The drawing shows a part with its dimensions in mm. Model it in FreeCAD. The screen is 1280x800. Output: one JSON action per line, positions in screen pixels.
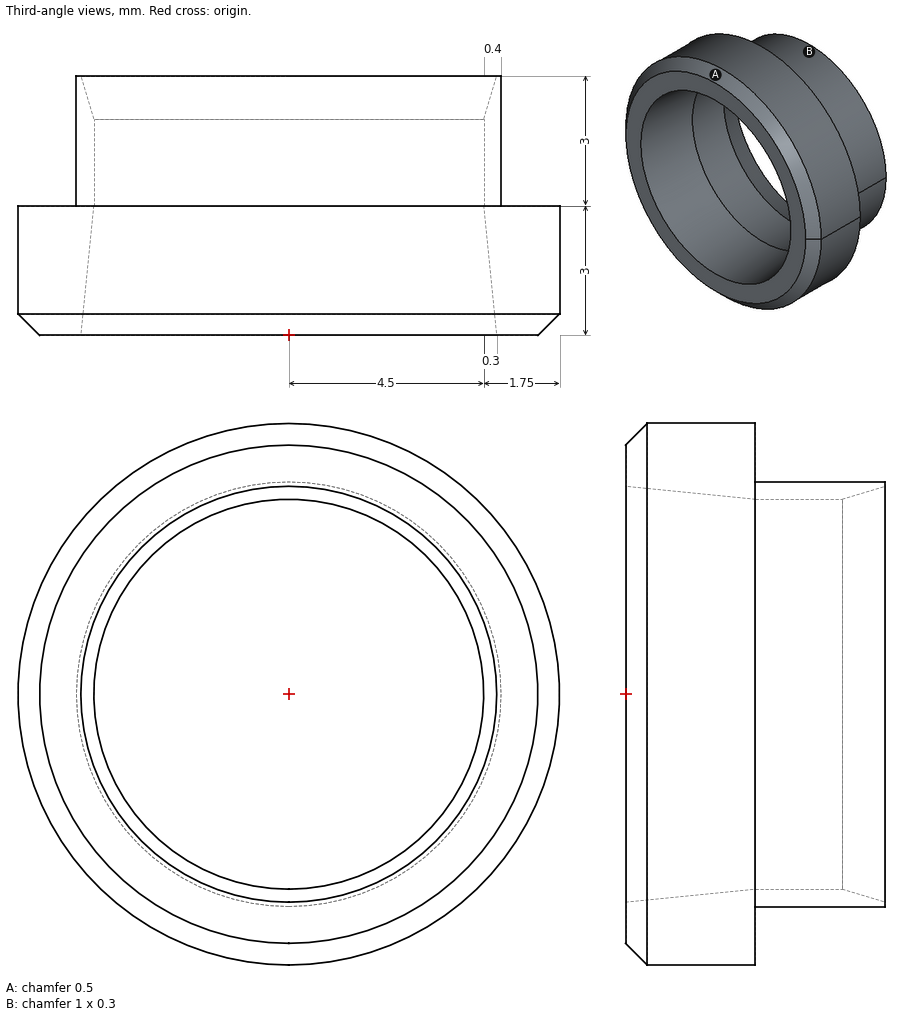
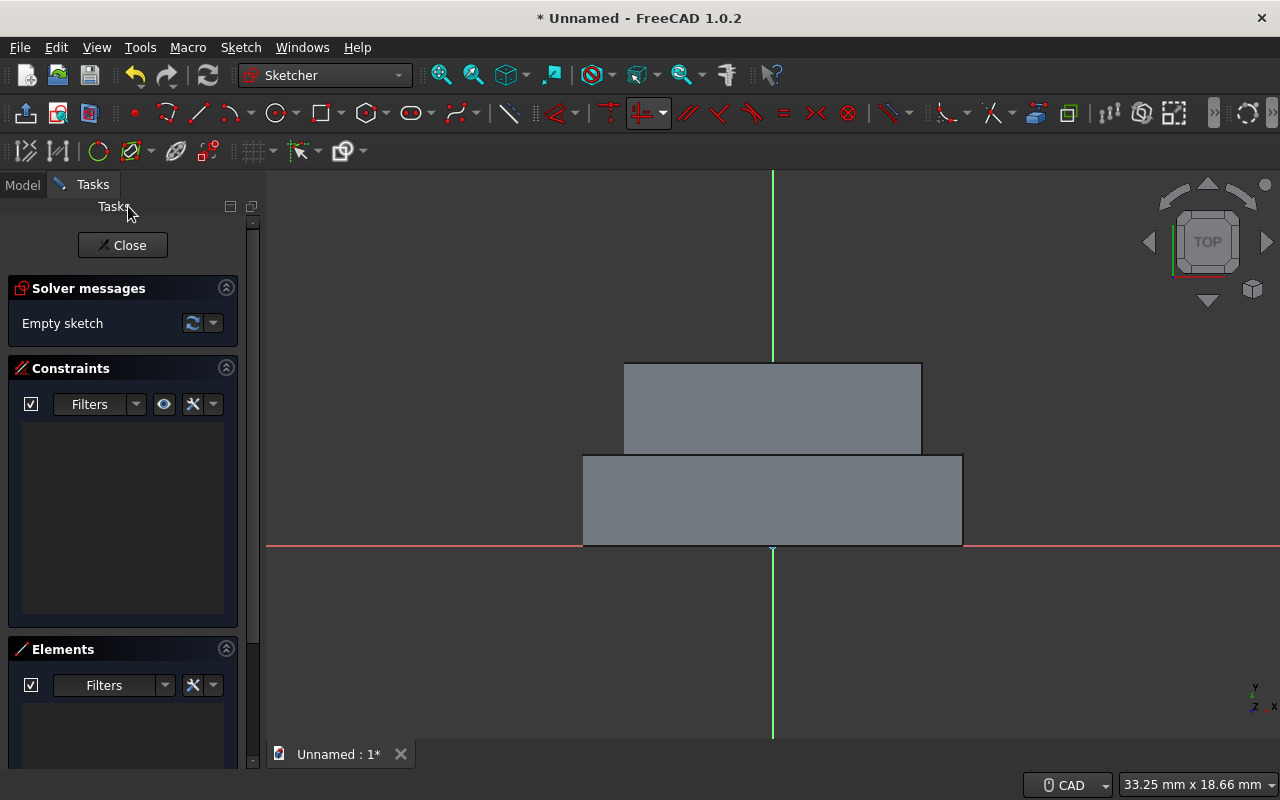
{"action": "left_click", "coordinate": [90, 114]}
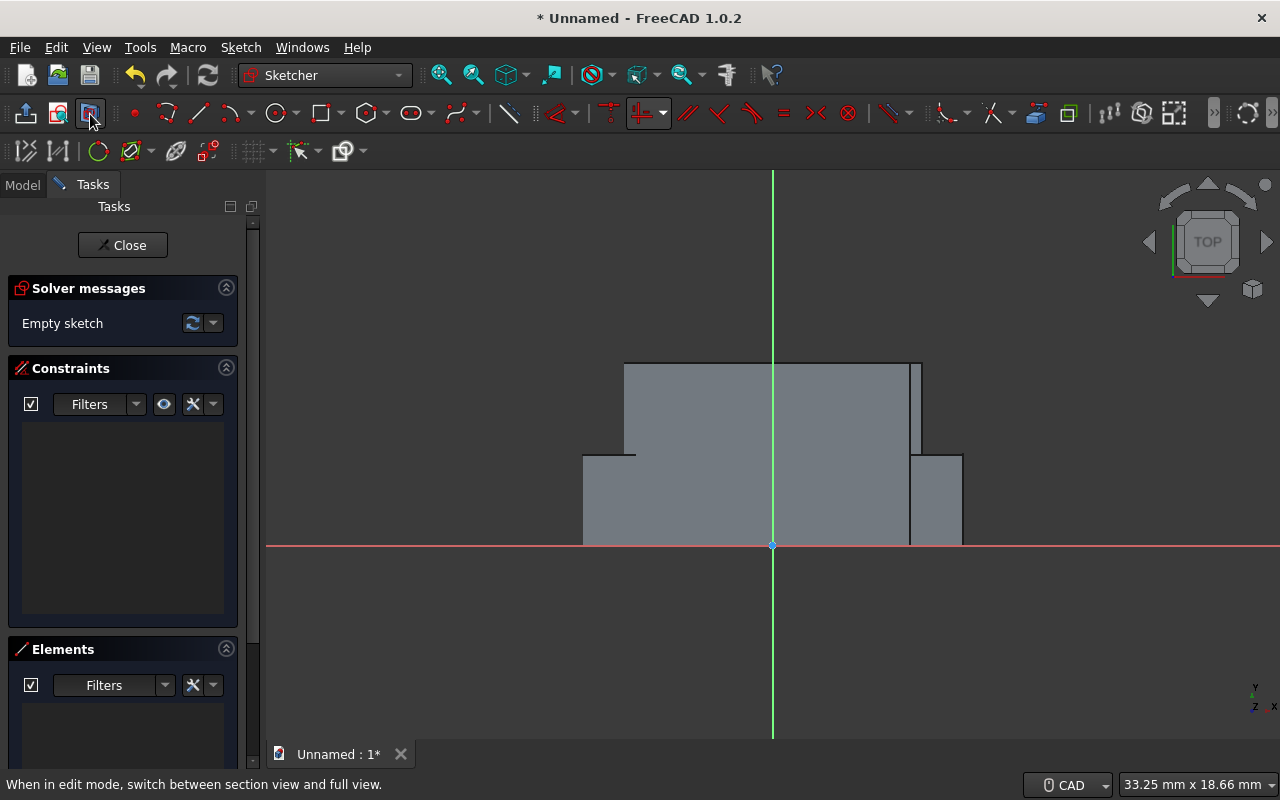
{"action": "scroll", "coordinate": [892, 515], "scroll_direction": "up", "scroll_amount": 7}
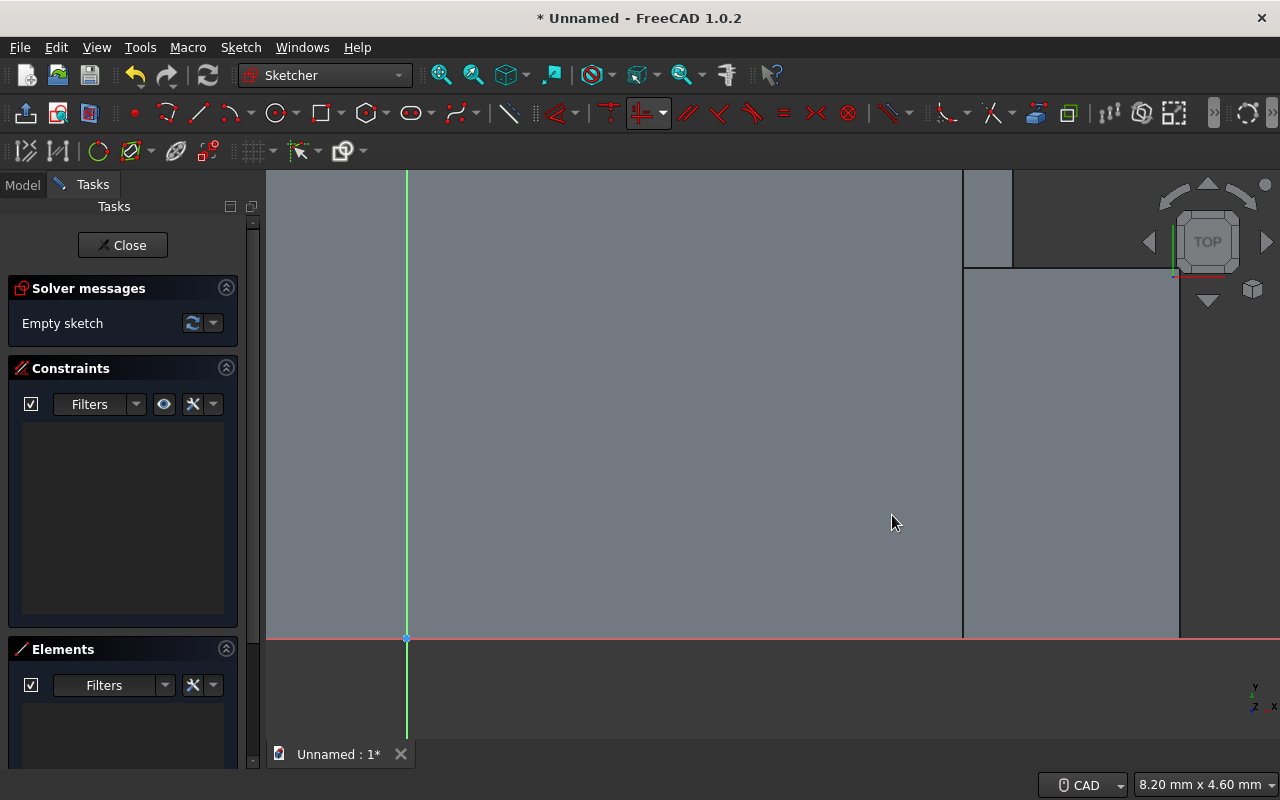
{"action": "key", "text": "g m"}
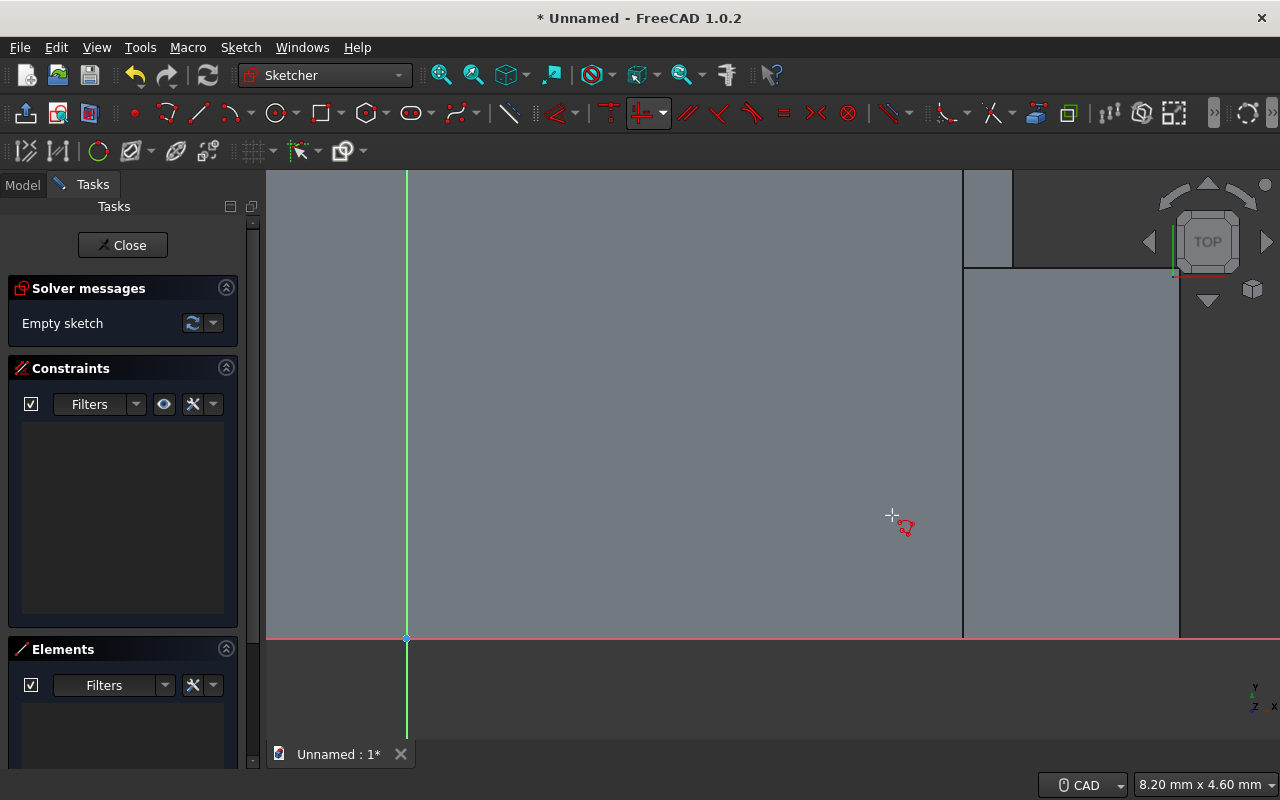
{"action": "left_click", "coordinate": [963, 639]}
{"action": "left_click", "coordinate": [1001, 630]}
{"action": "left_click", "coordinate": [963, 268]}
{"action": "left_click", "coordinate": [963, 639]}
{"action": "key", "text": "Escape"}
{"action": "key", "text": "Escape"}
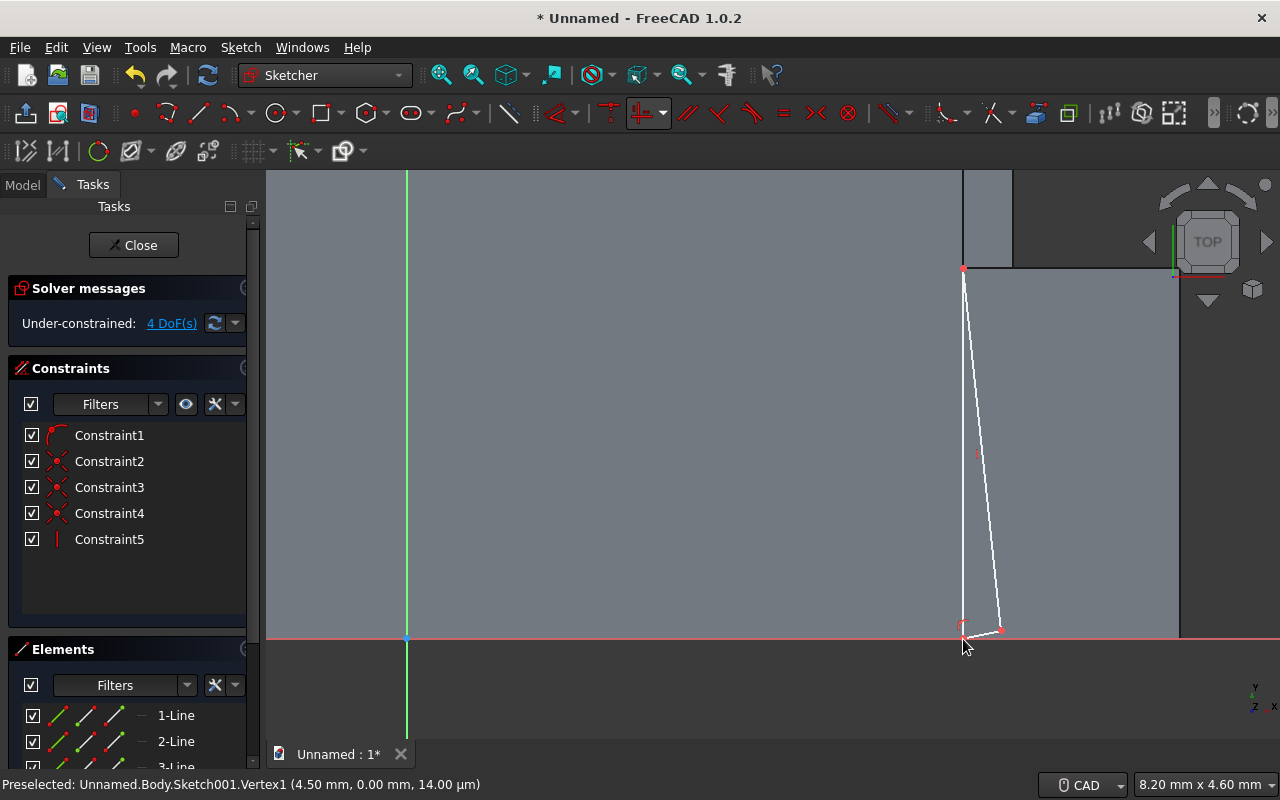
{"action": "left_click", "coordinate": [974, 636]}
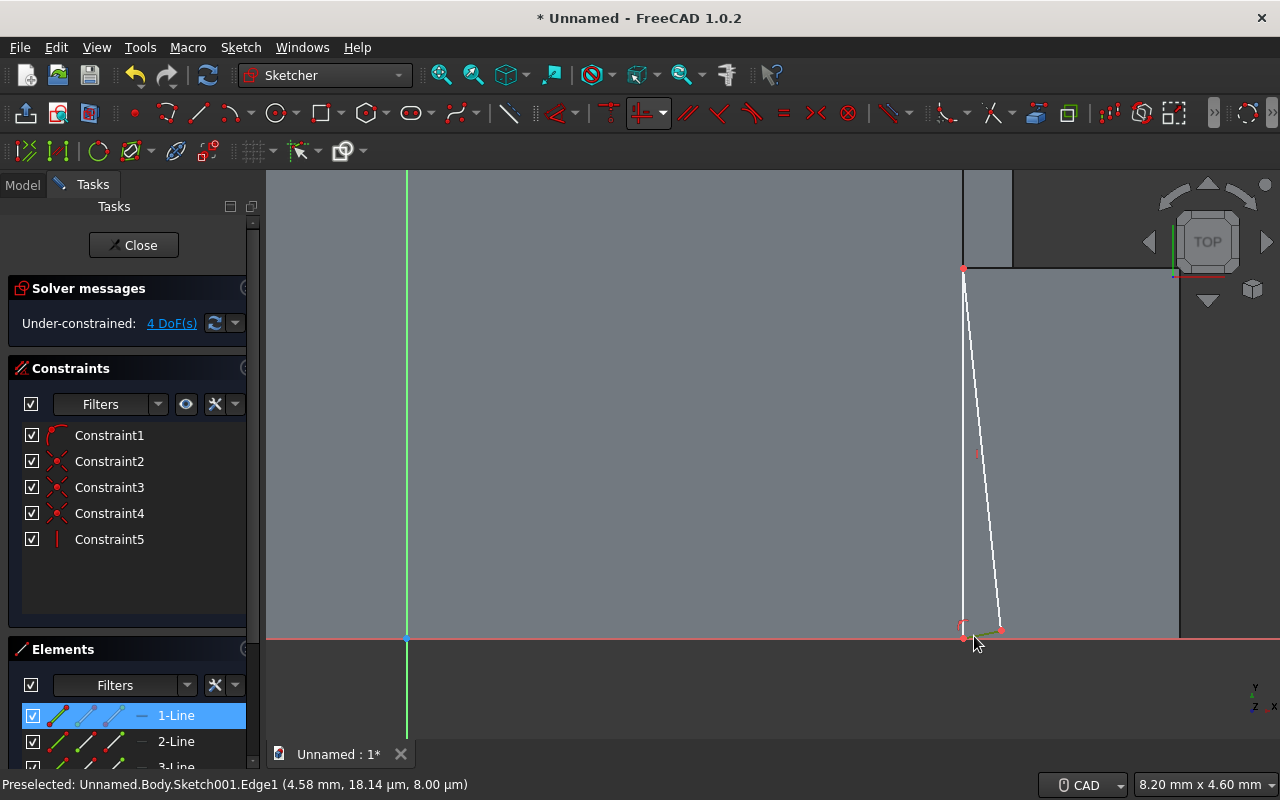
{"action": "key", "text": "h"}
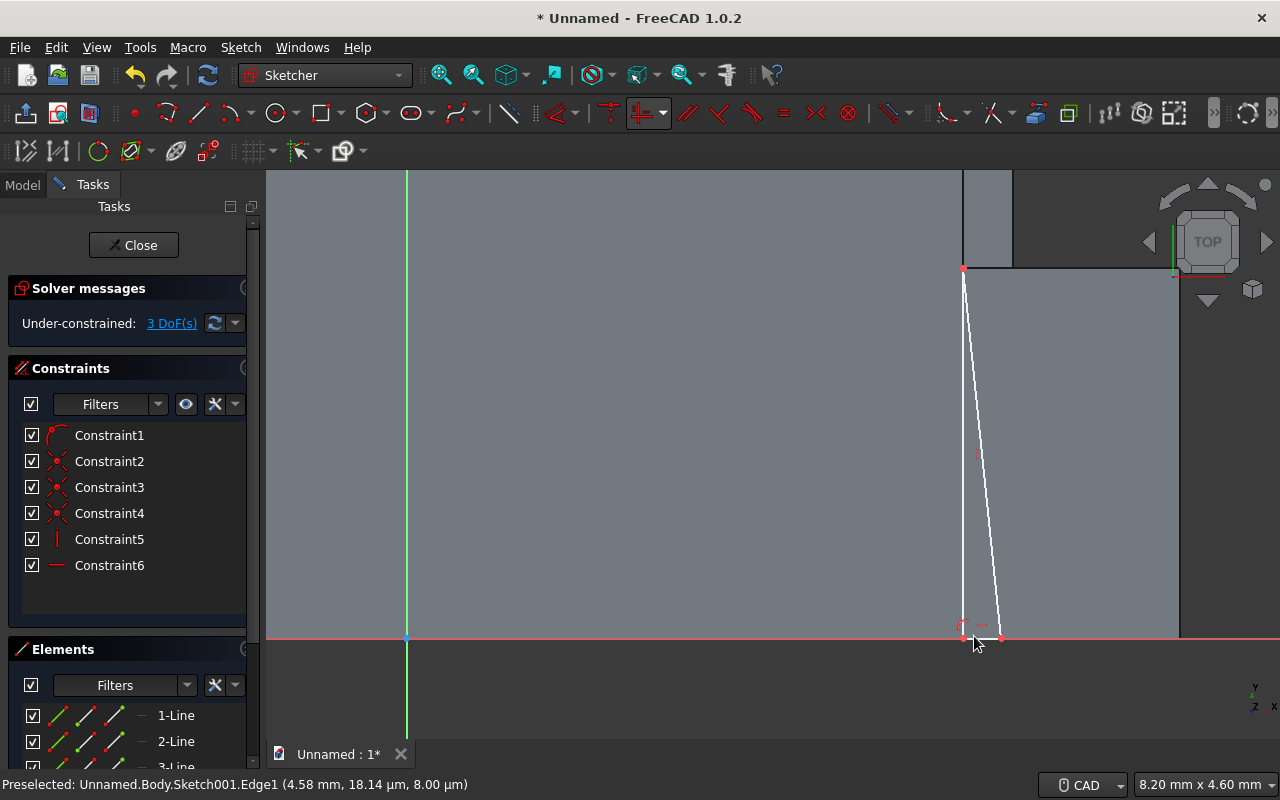
{"action": "left_click", "coordinate": [556, 114]}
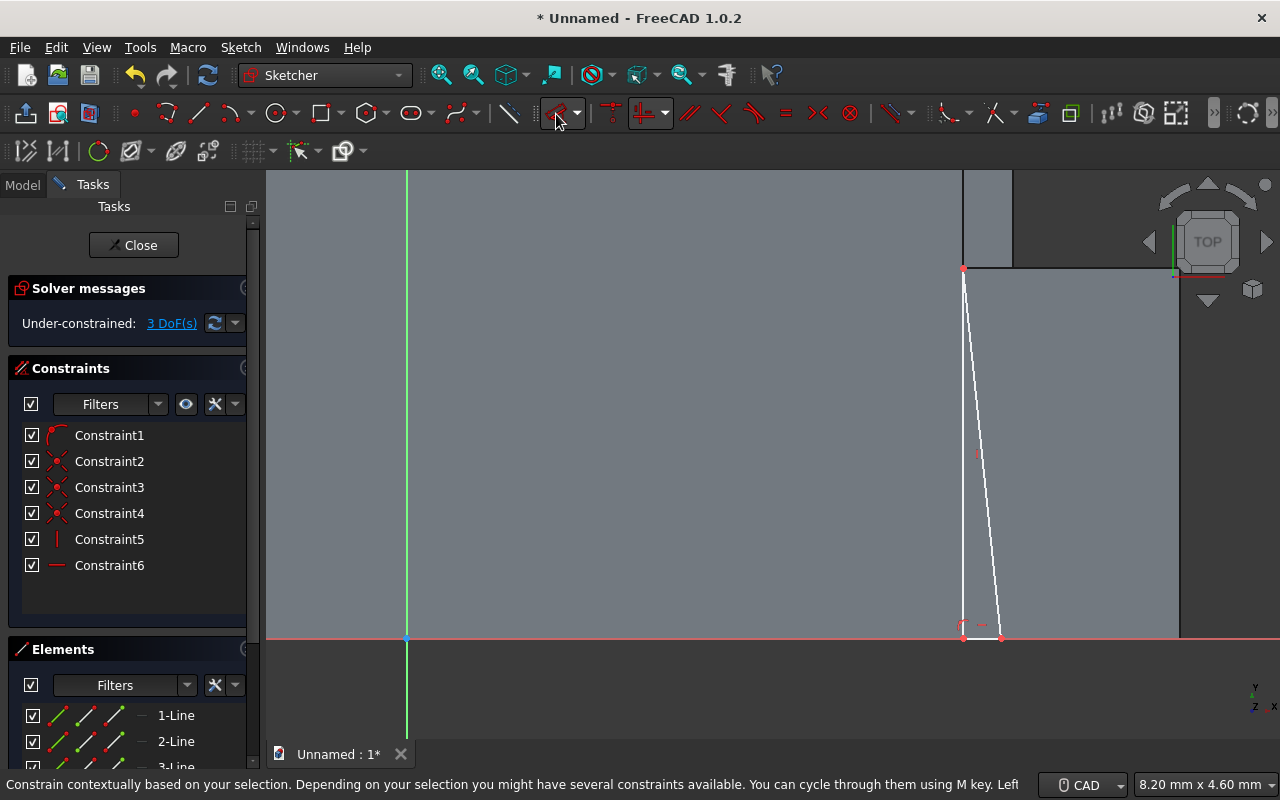
{"action": "left_click", "coordinate": [963, 380]}
{"action": "left_click", "coordinate": [997, 454]}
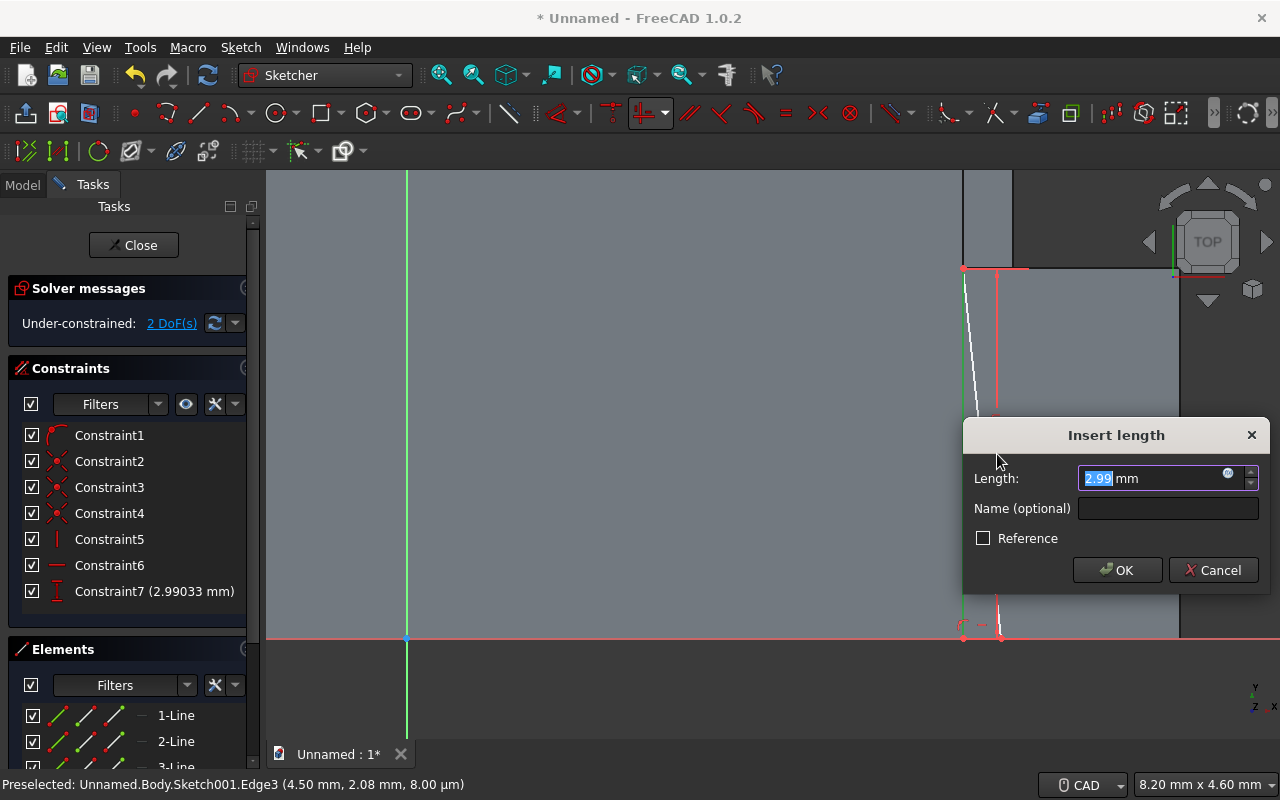
{"action": "type", "text": "3"}
{"action": "key", "text": "Return"}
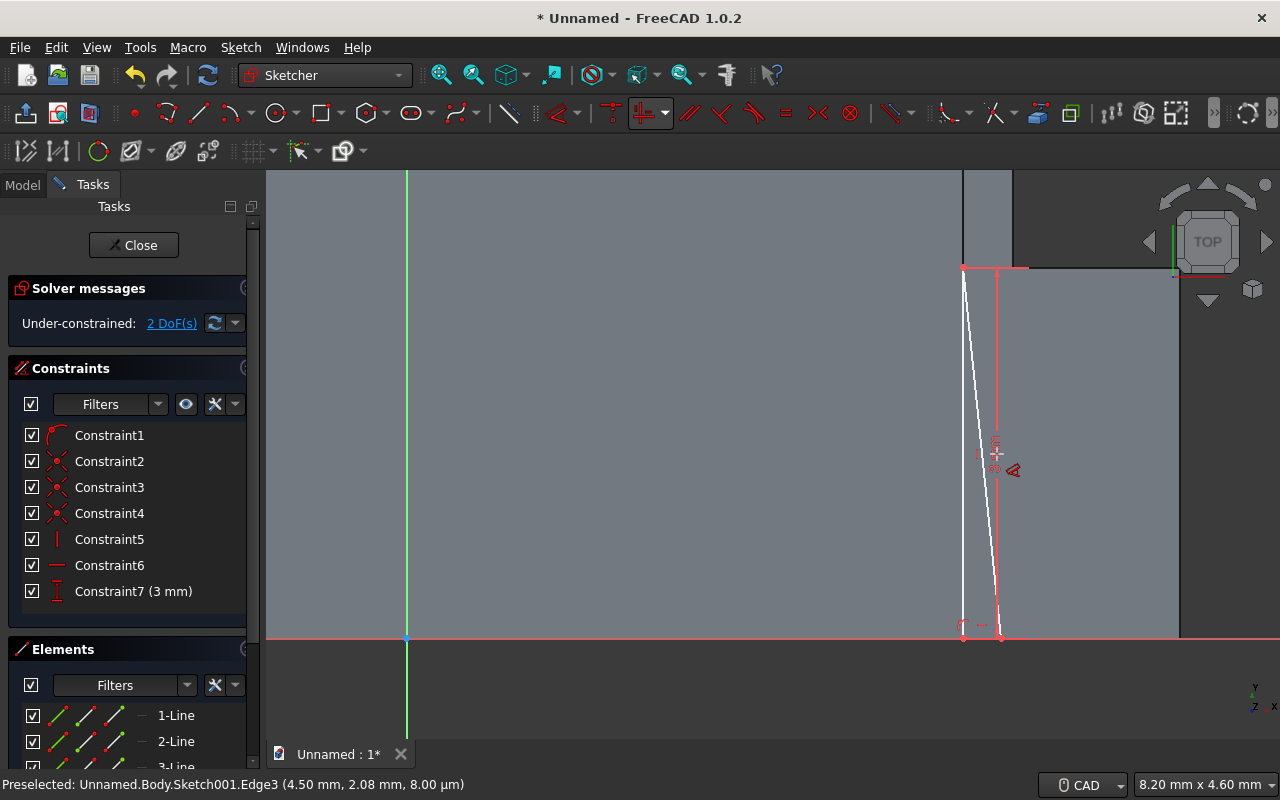
{"action": "left_click", "coordinate": [974, 639]}
{"action": "left_click", "coordinate": [982, 673]}